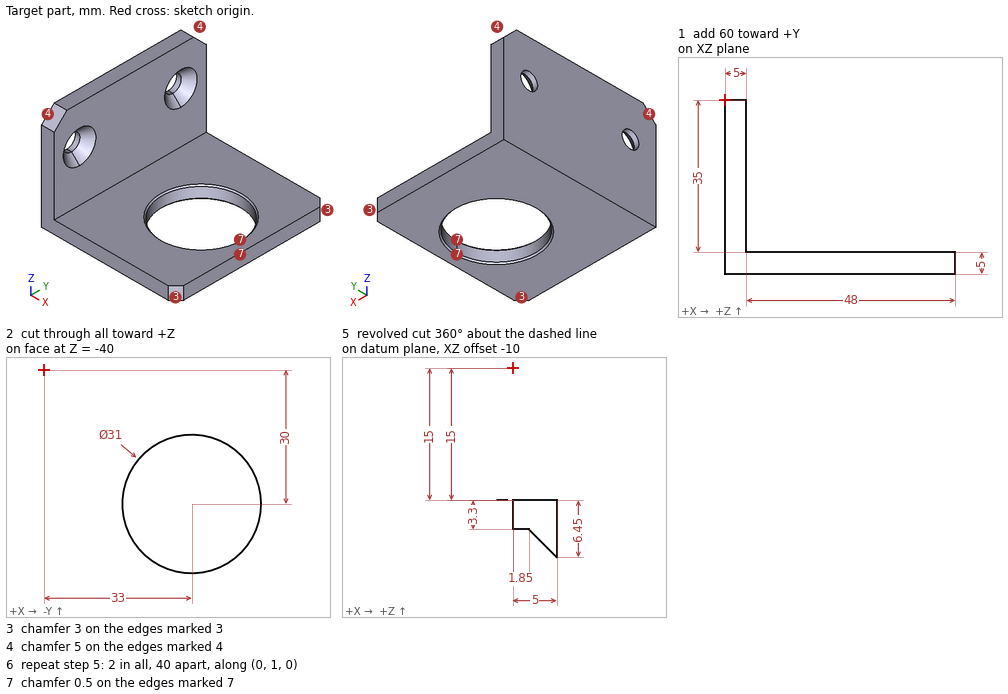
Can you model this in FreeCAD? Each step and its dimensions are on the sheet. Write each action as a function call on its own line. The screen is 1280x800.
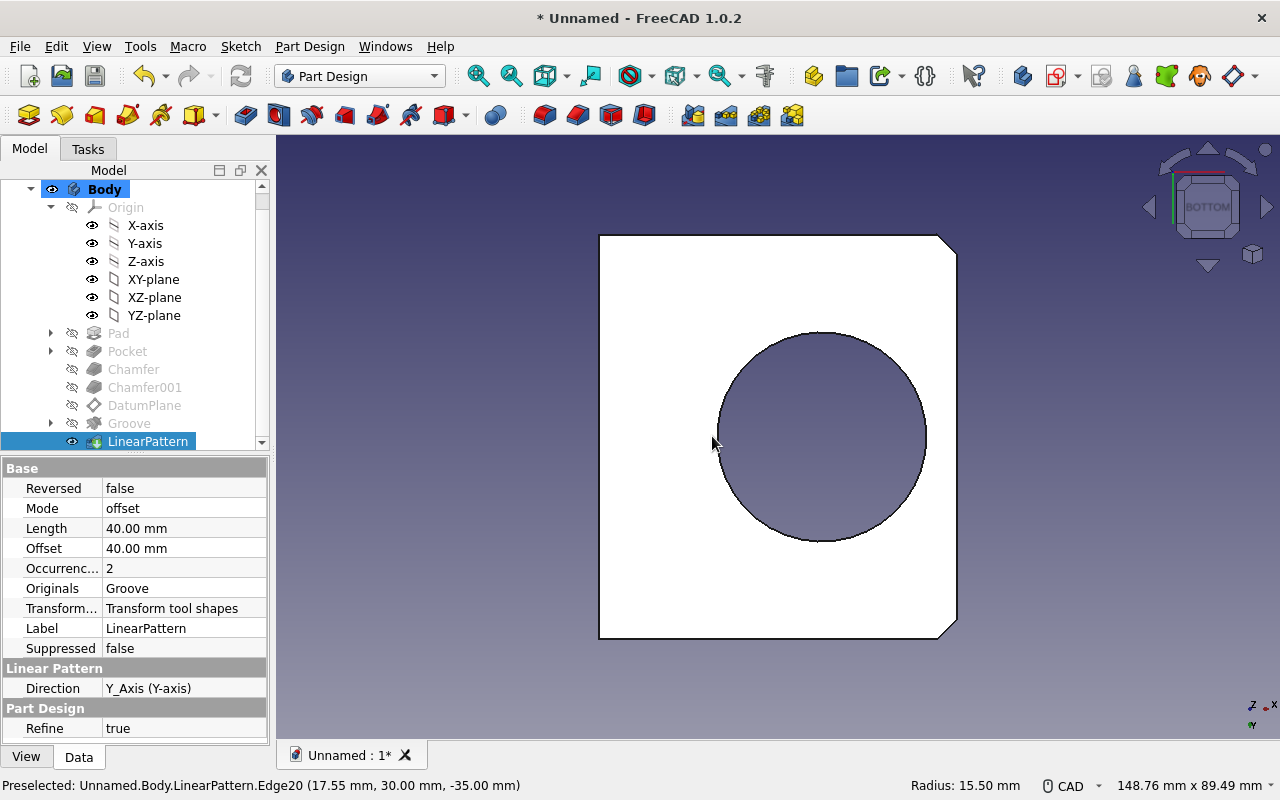
click(717, 436, ctrl)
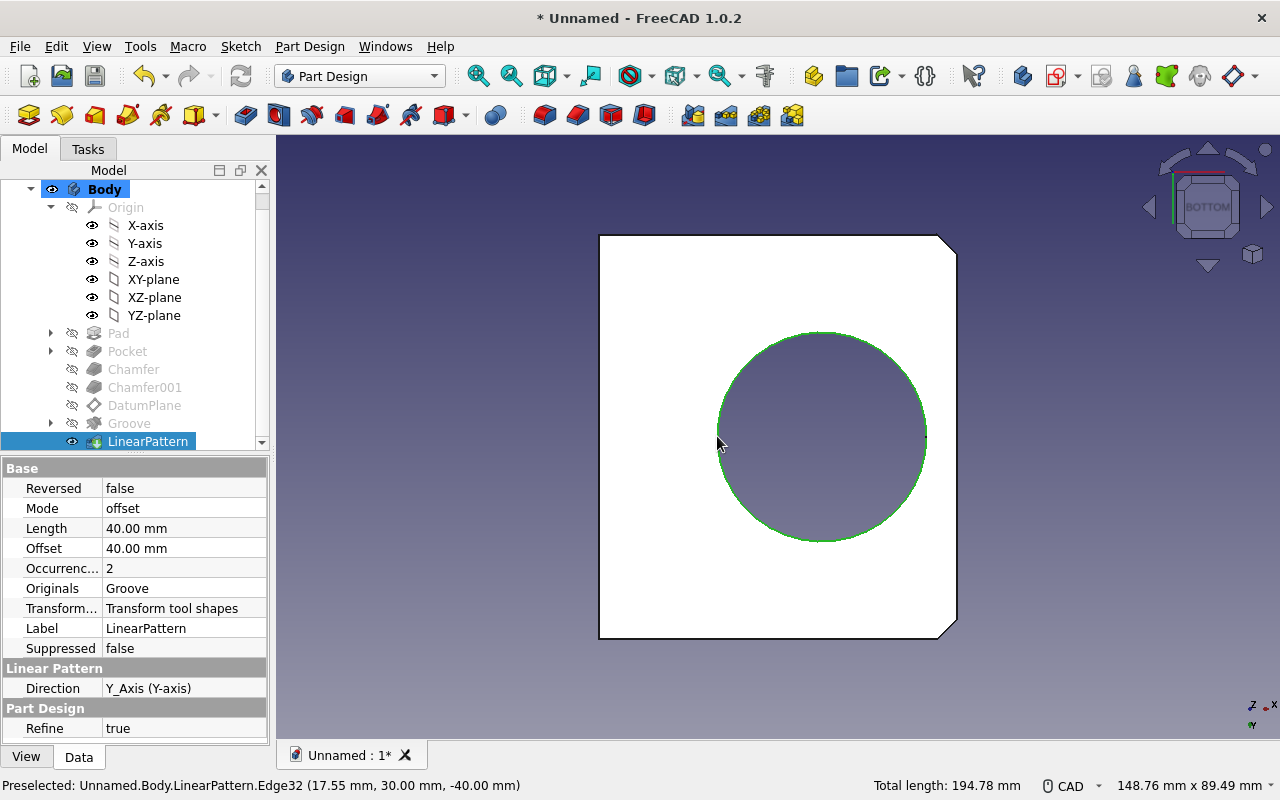
click(578, 116)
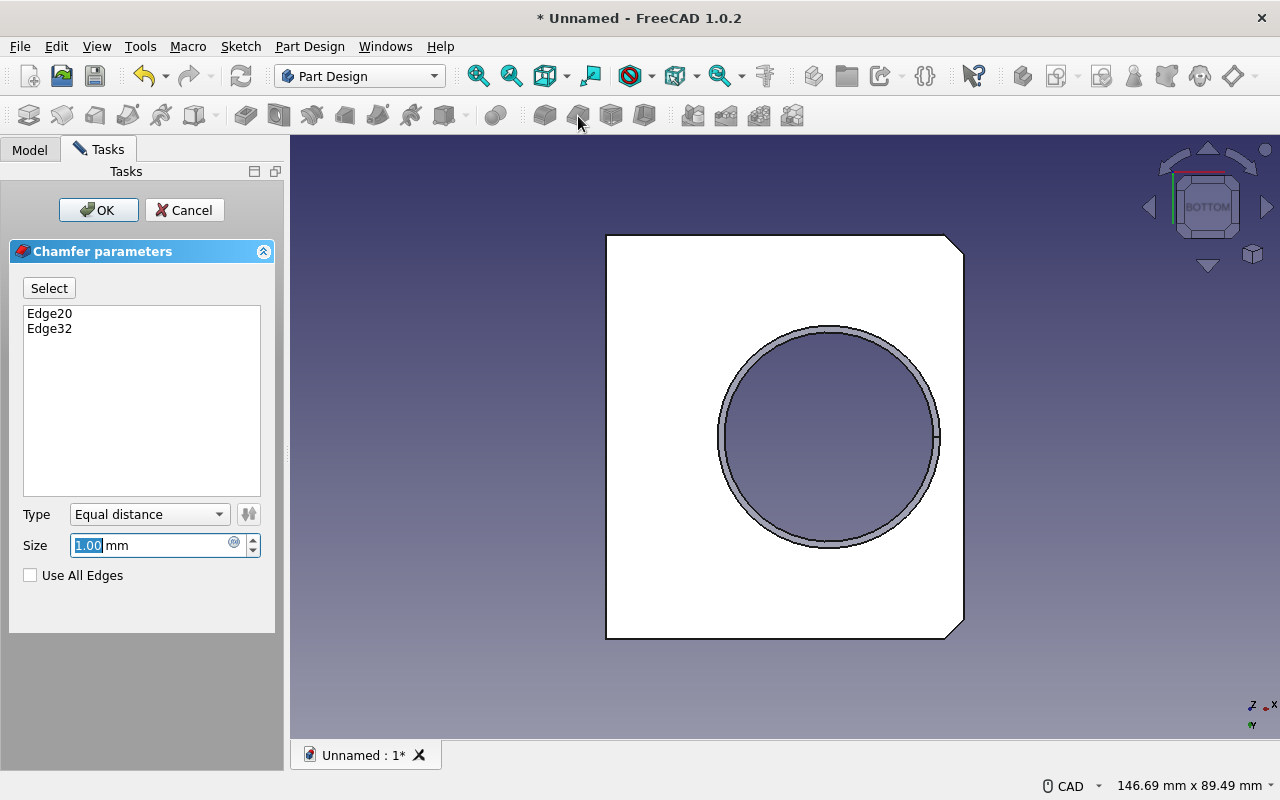
text(0.5)
key(Tab)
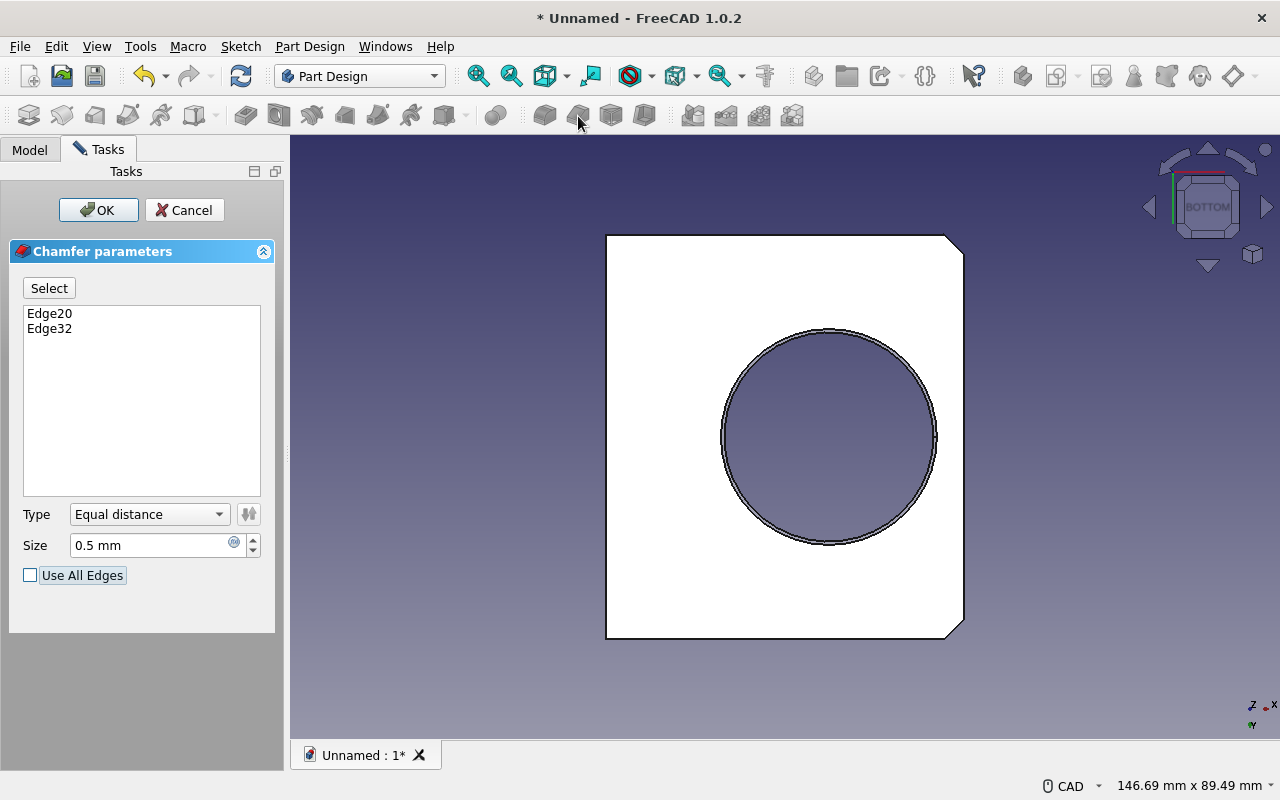
click(99, 210)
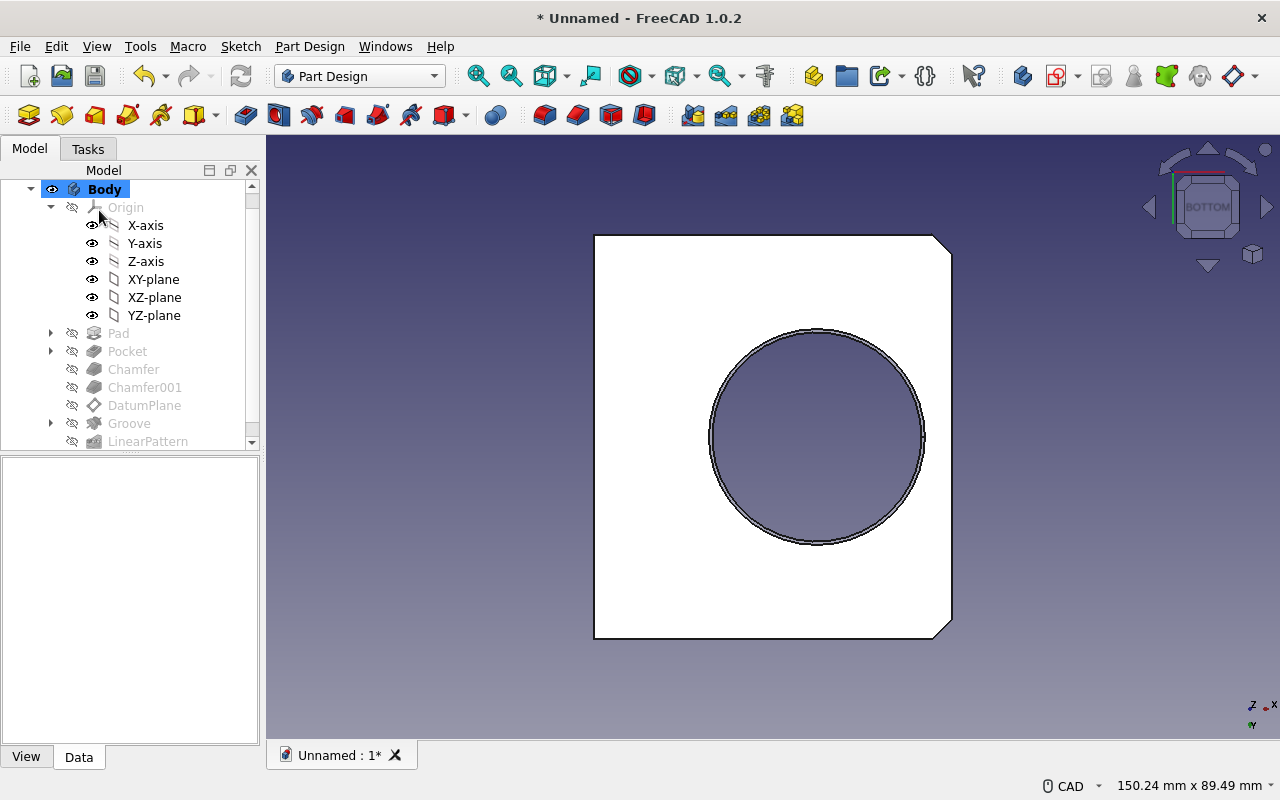
key(0)